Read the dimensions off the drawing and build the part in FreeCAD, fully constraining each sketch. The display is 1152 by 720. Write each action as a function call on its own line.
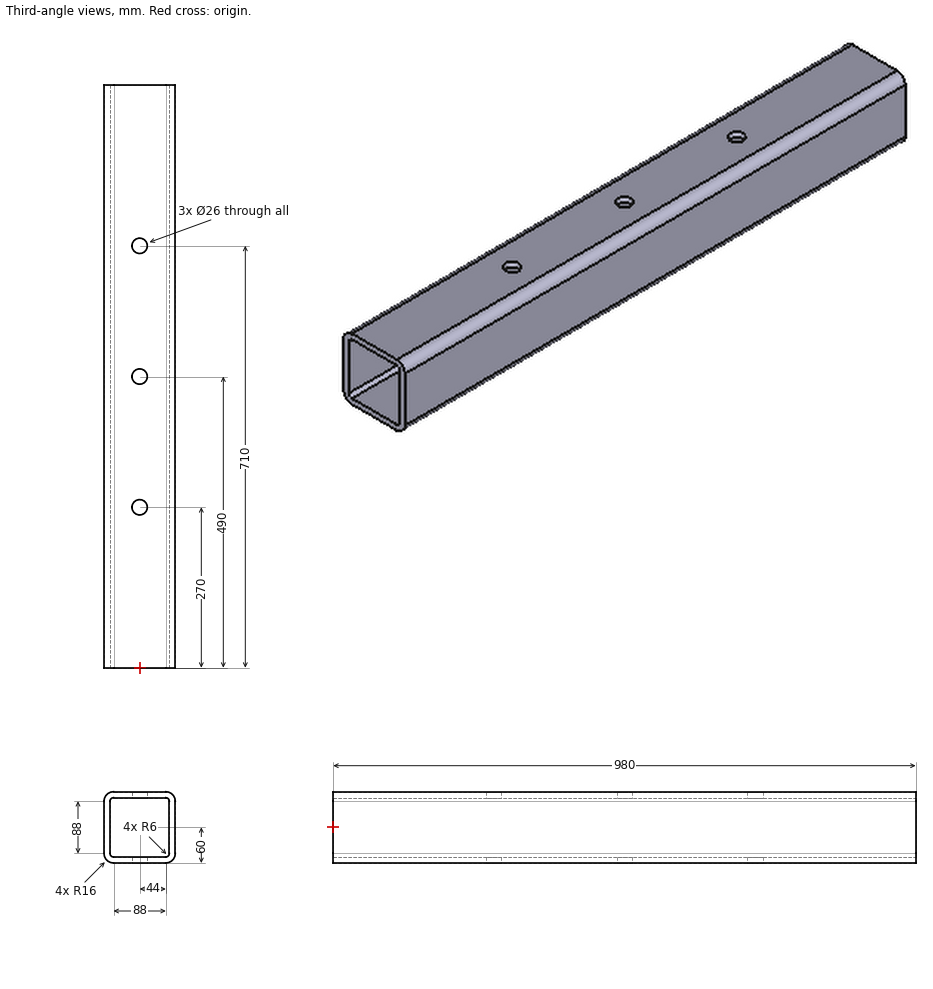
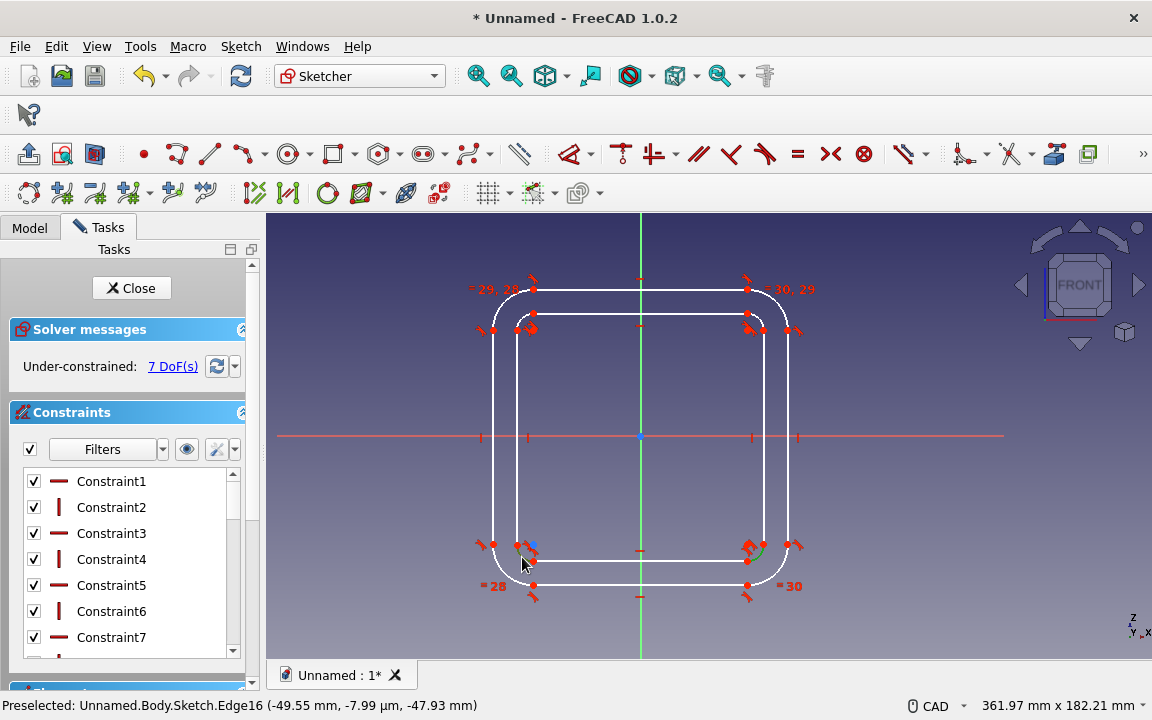
click(798, 154)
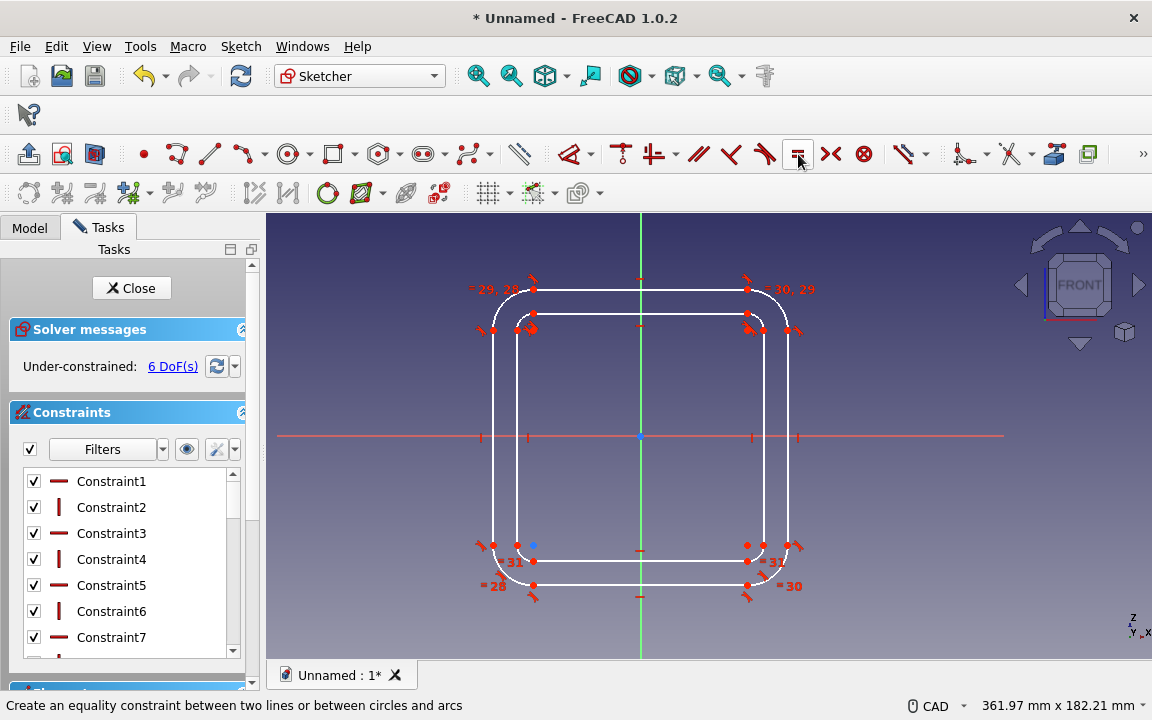
click(495, 558)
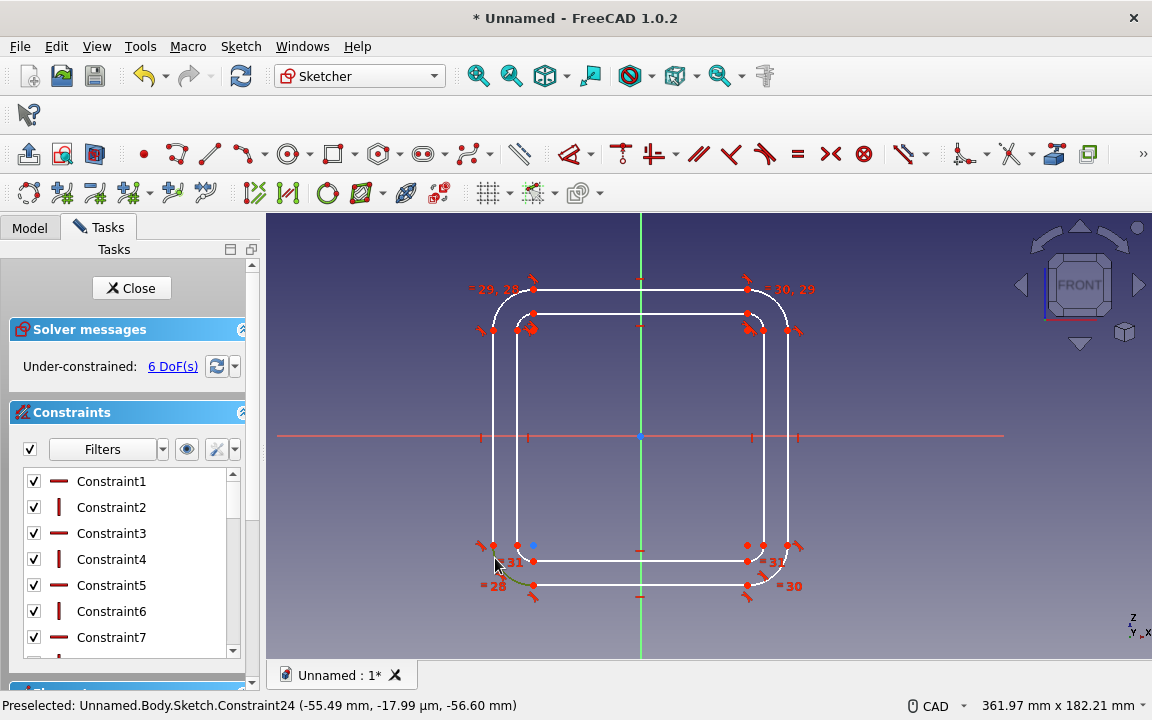
click(590, 154)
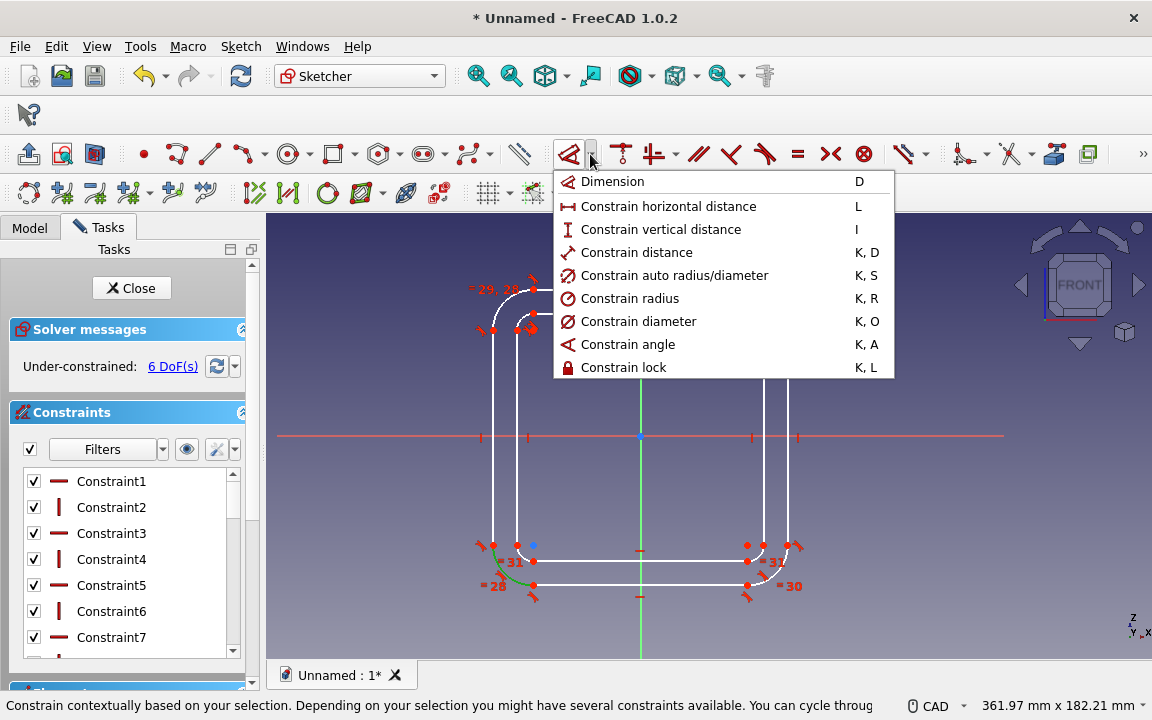
click(724, 298)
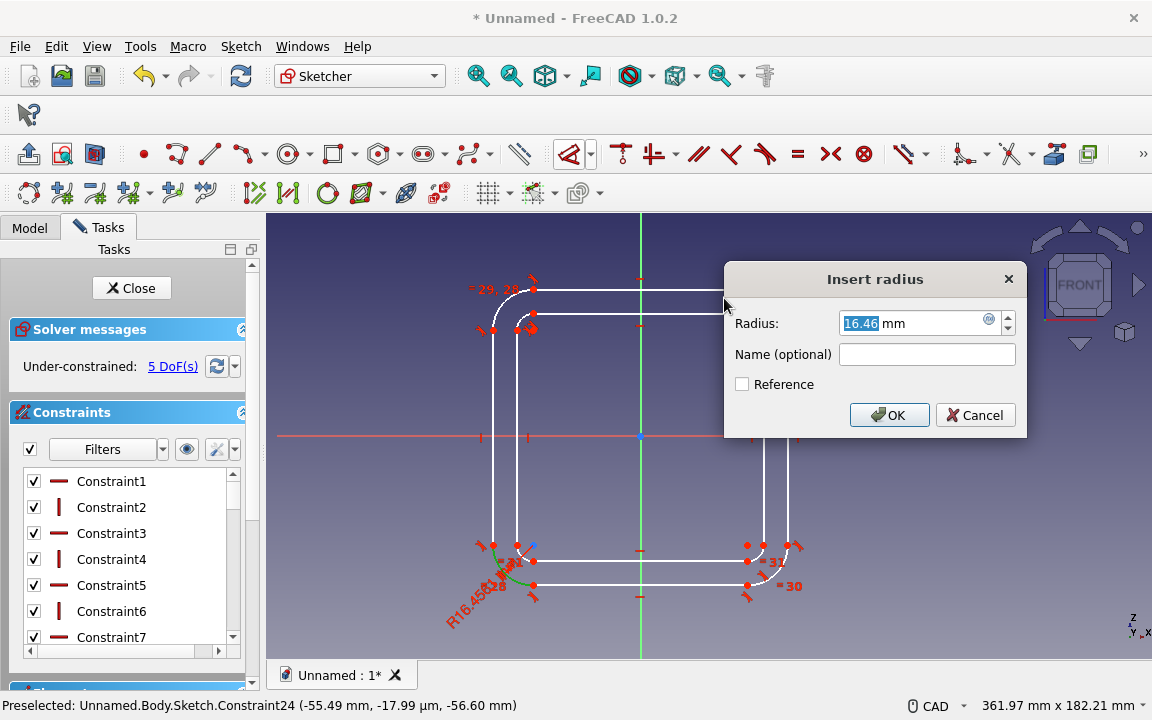
text(16)
key(Return)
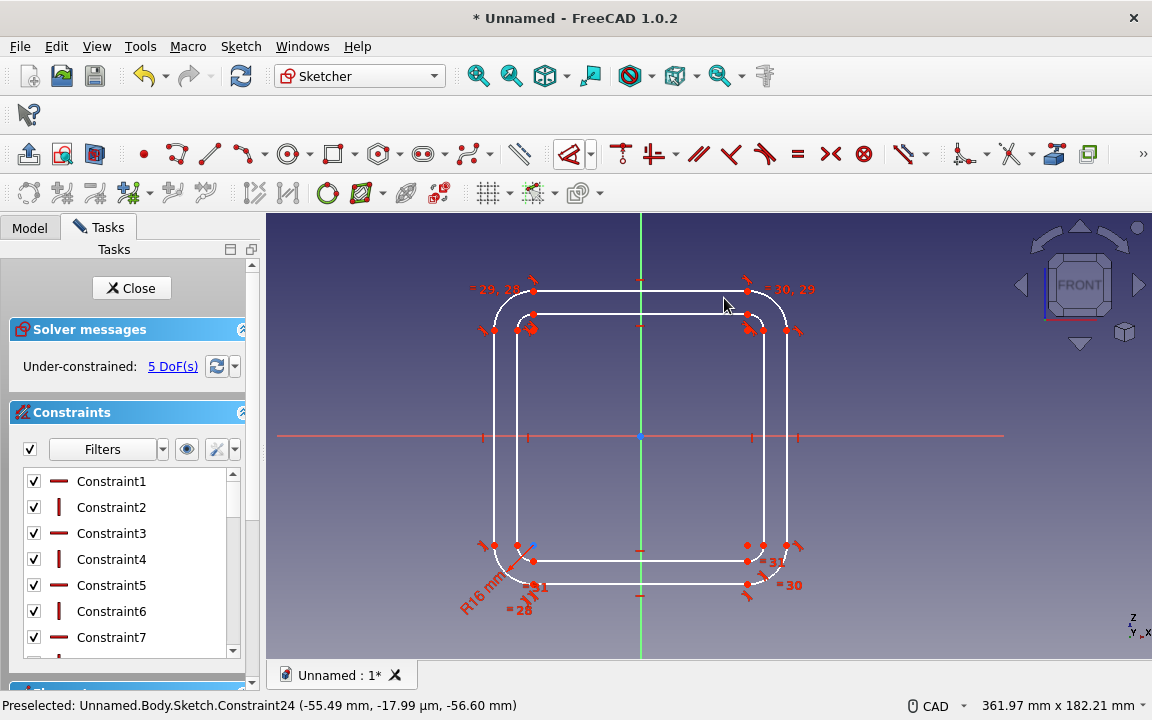
scroll(759, 557, up, 5)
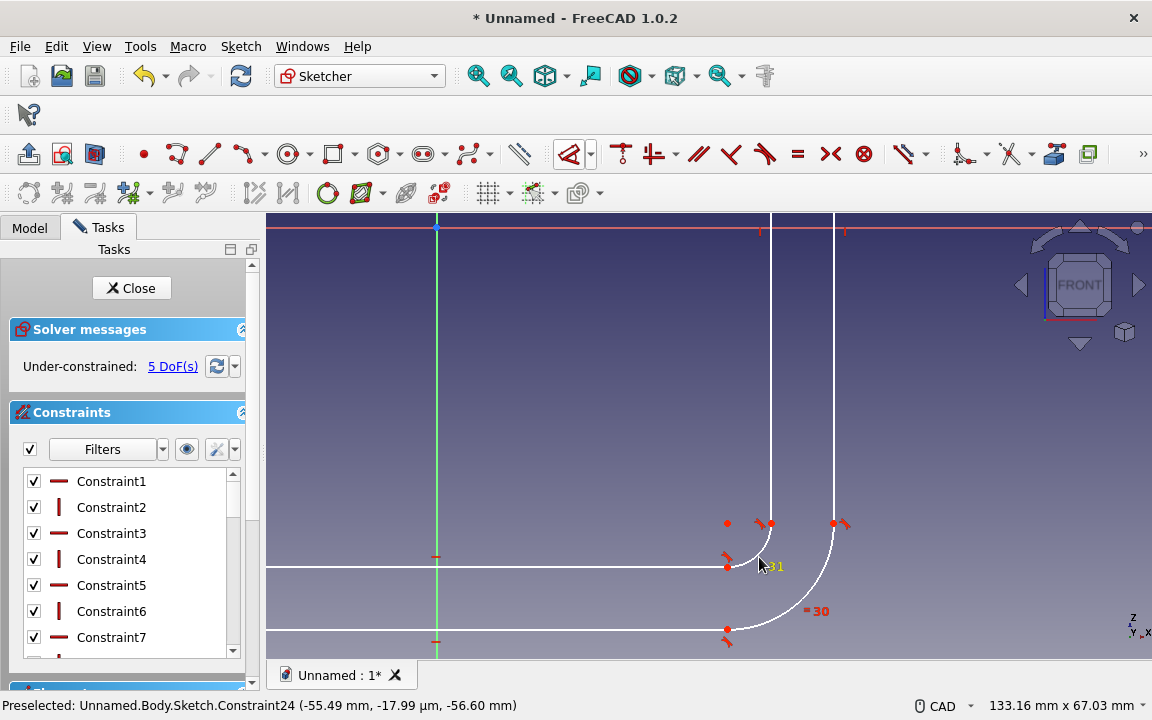
click(758, 554)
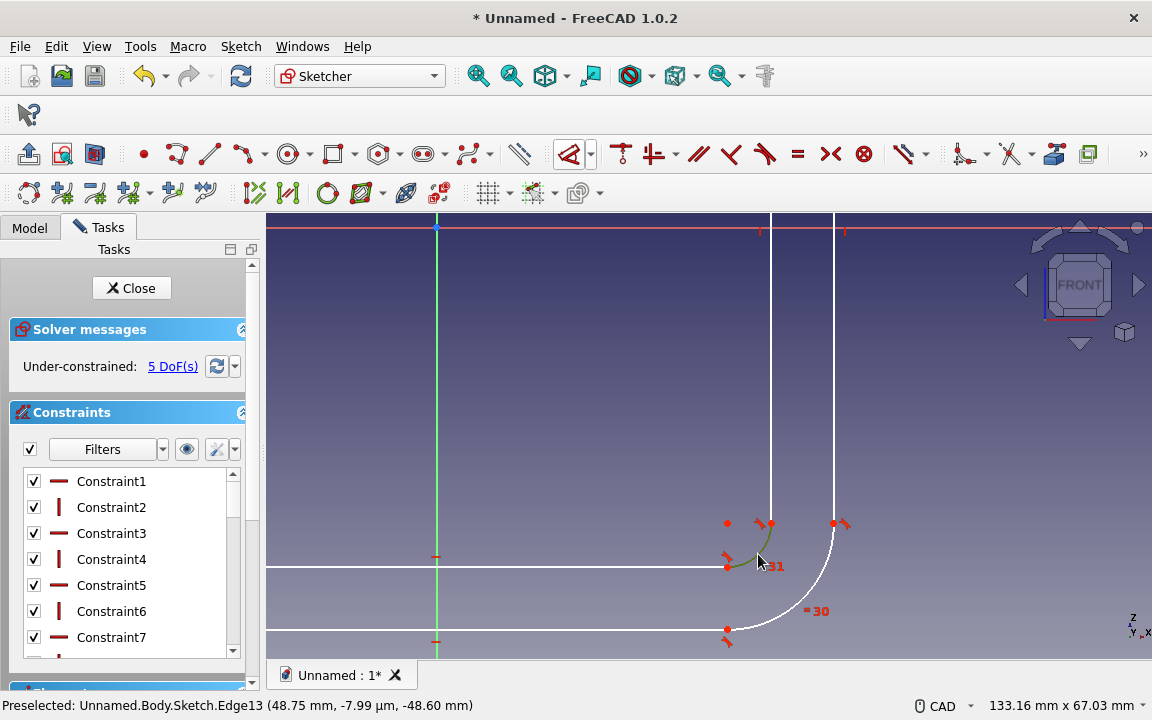
key(k)
key(r)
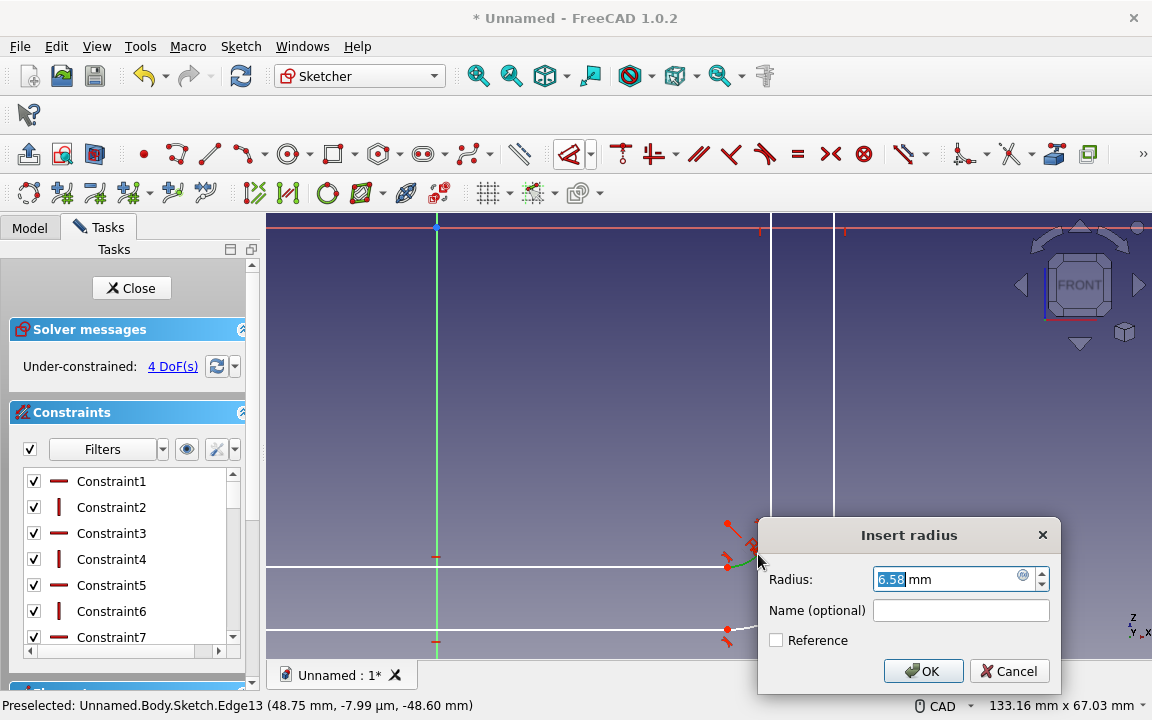
text(6)
key(Return)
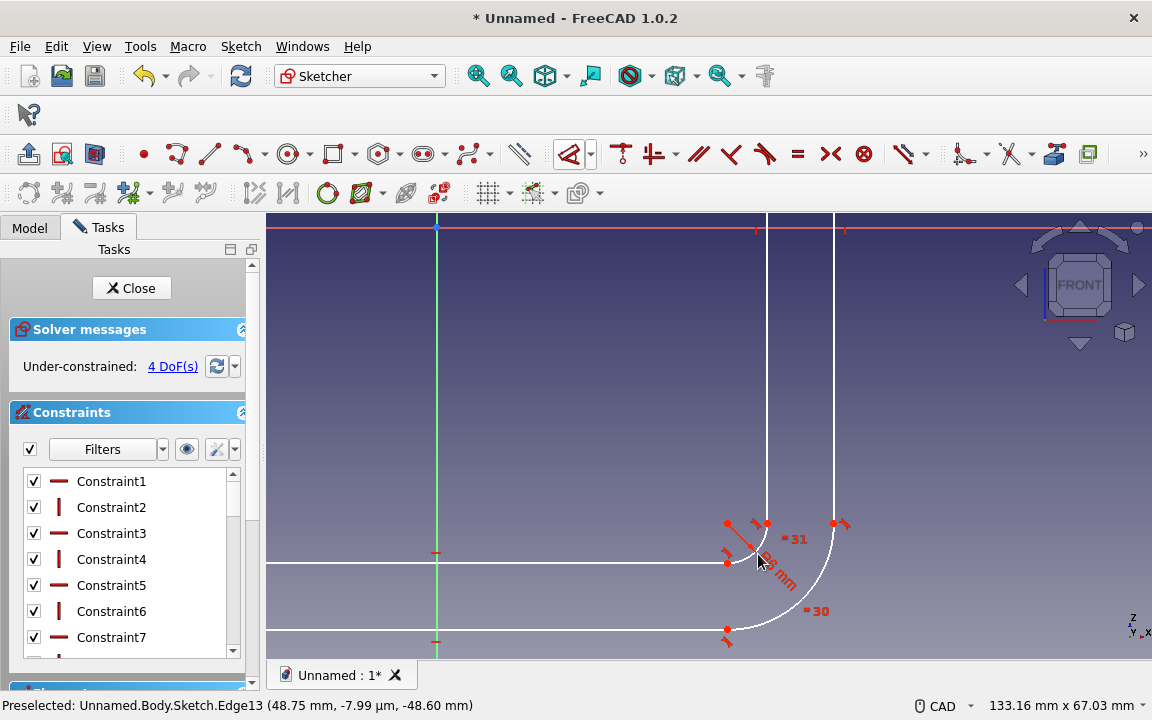
click(553, 630)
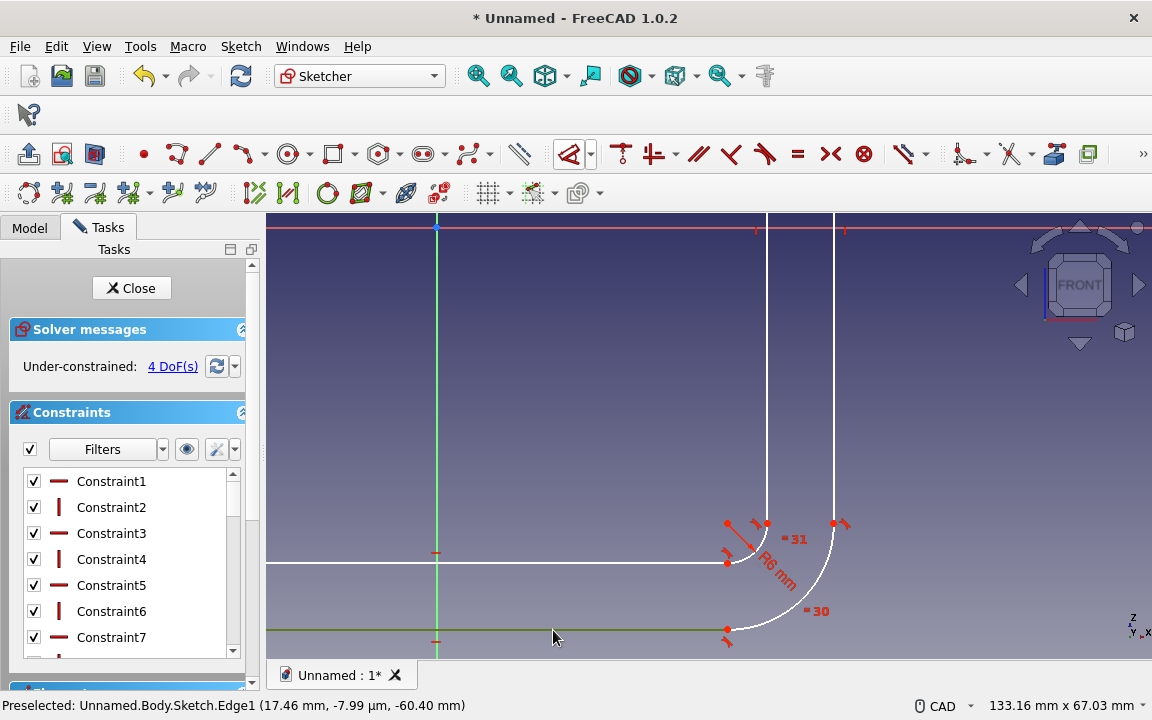
click(590, 154)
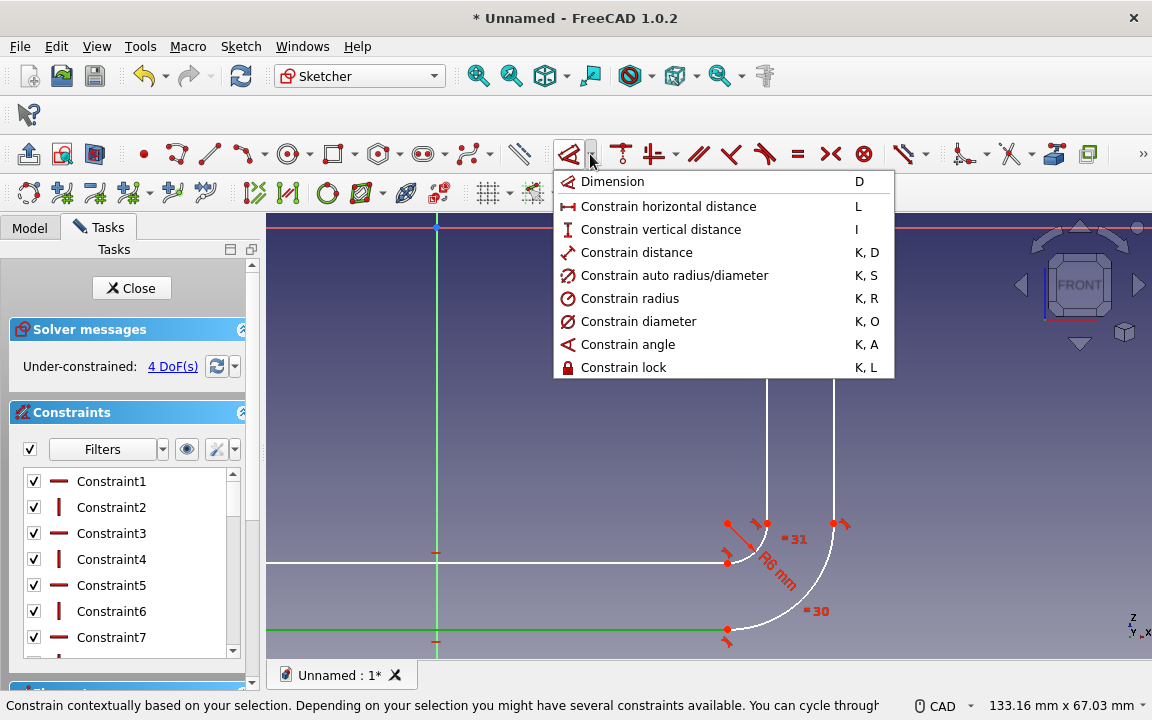
click(724, 206)